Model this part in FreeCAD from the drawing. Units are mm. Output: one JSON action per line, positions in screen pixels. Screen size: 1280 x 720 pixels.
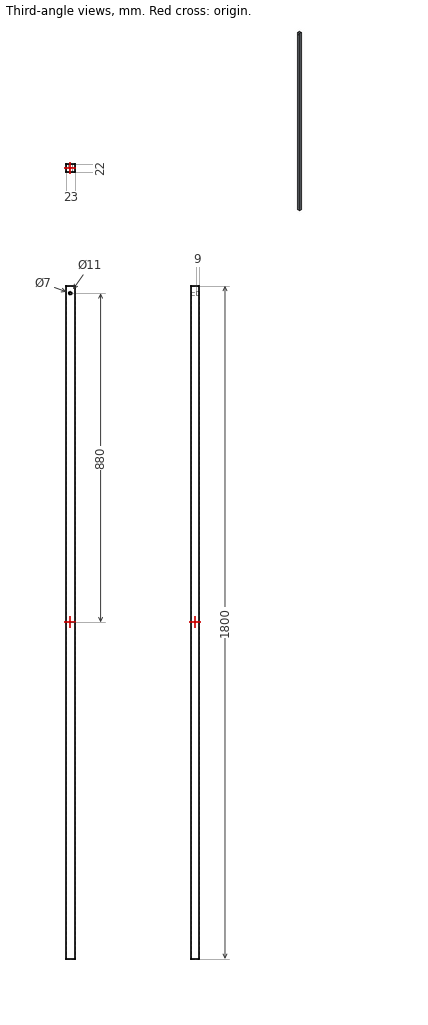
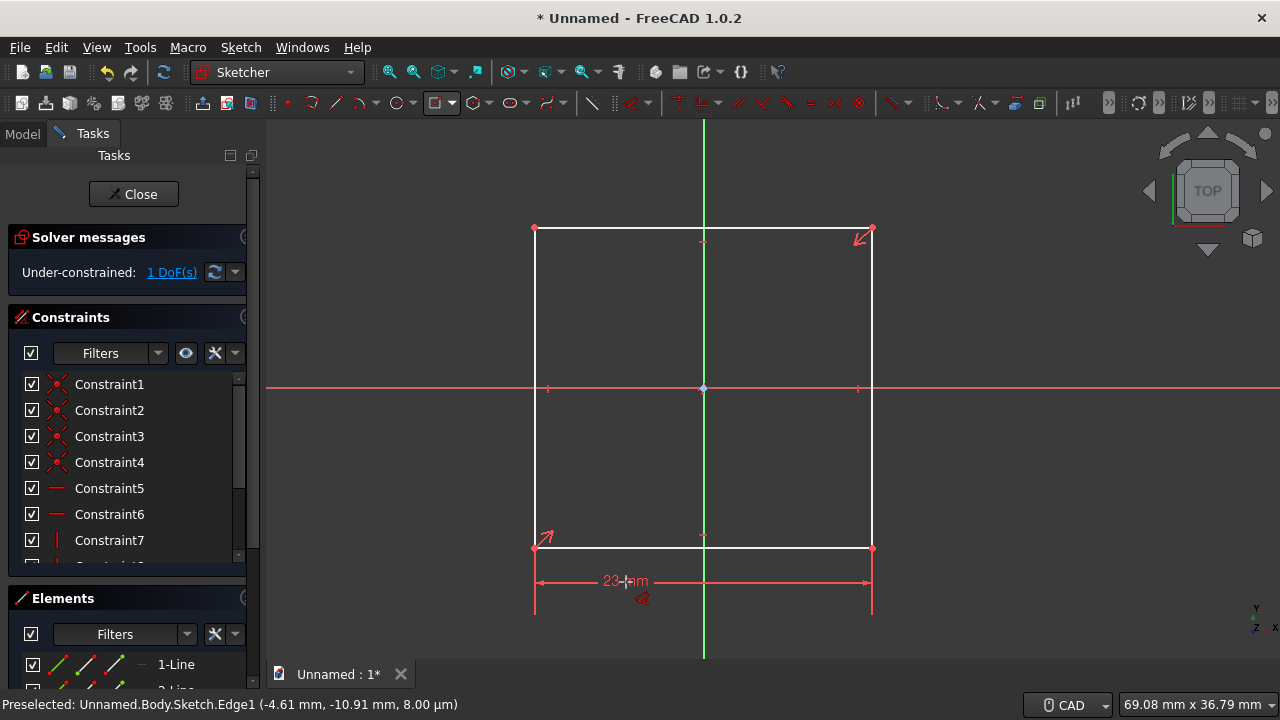
{"action": "left_click", "coordinate": [872, 452]}
{"action": "left_click", "coordinate": [906, 314]}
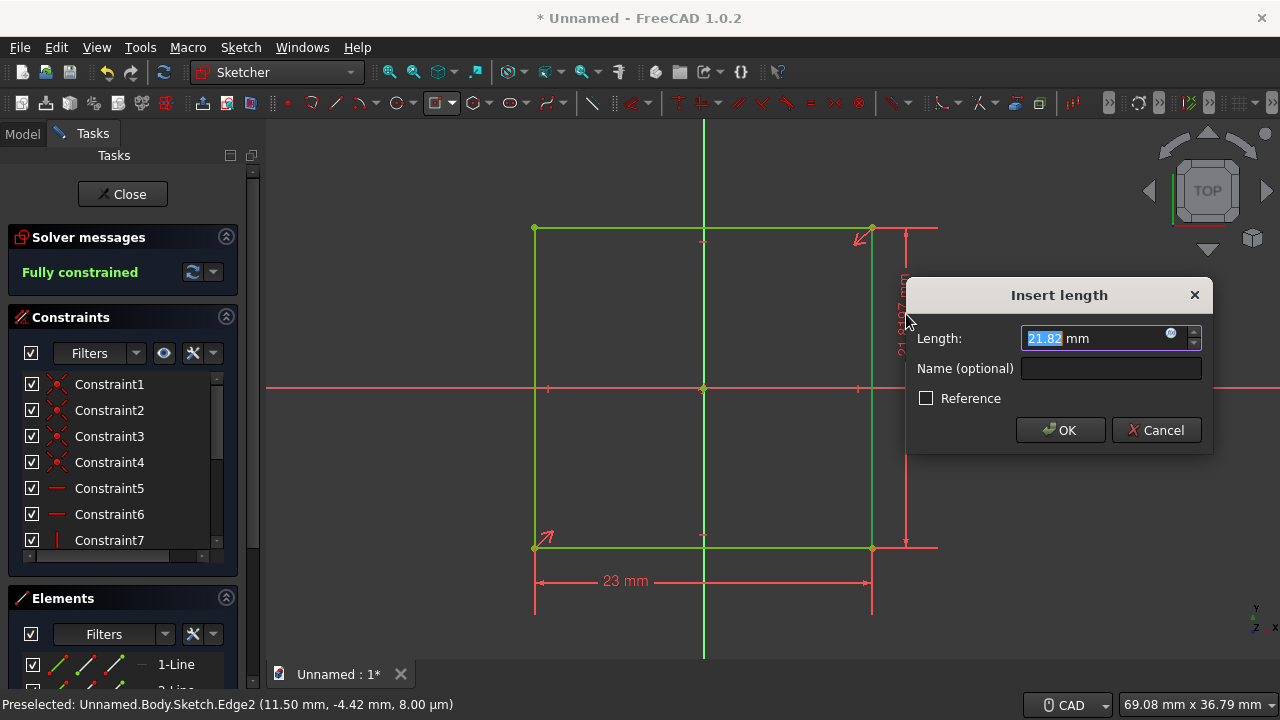
{"action": "type", "text": "22"}
{"action": "key", "text": "Return"}
{"action": "key", "text": "Escape"}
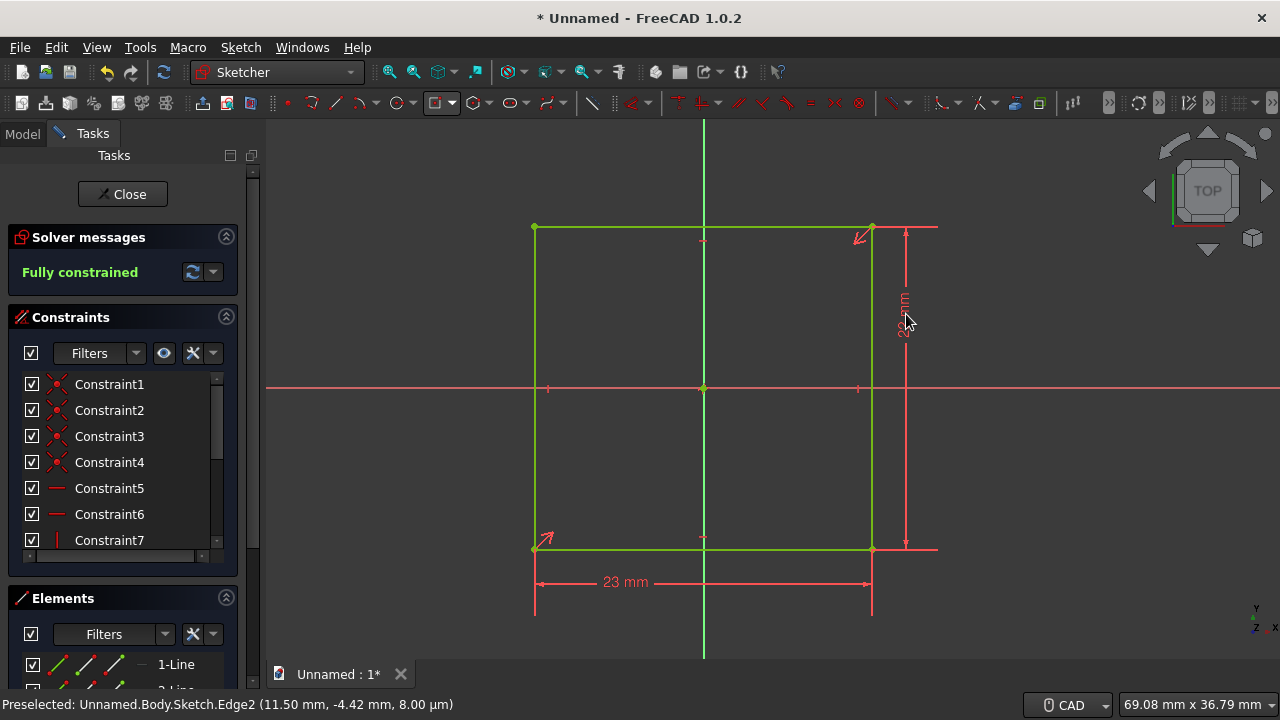
{"action": "left_click", "coordinate": [123, 194]}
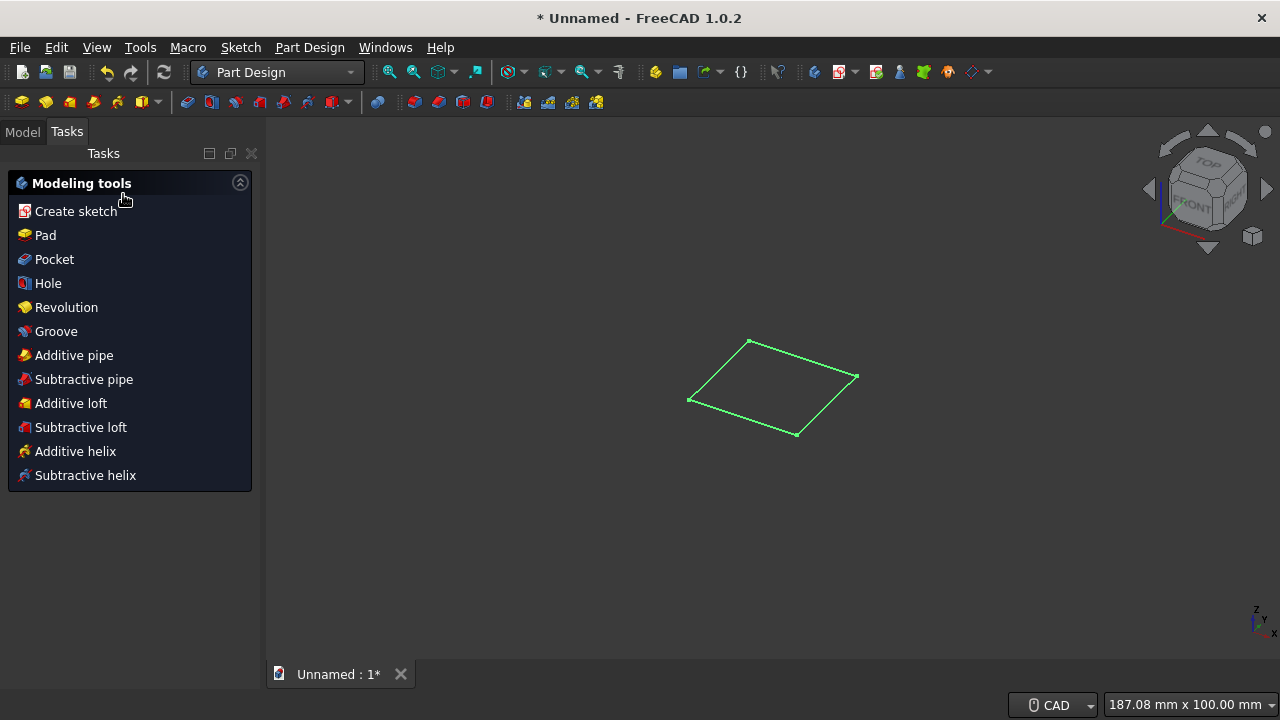
{"action": "left_click", "coordinate": [22, 102]}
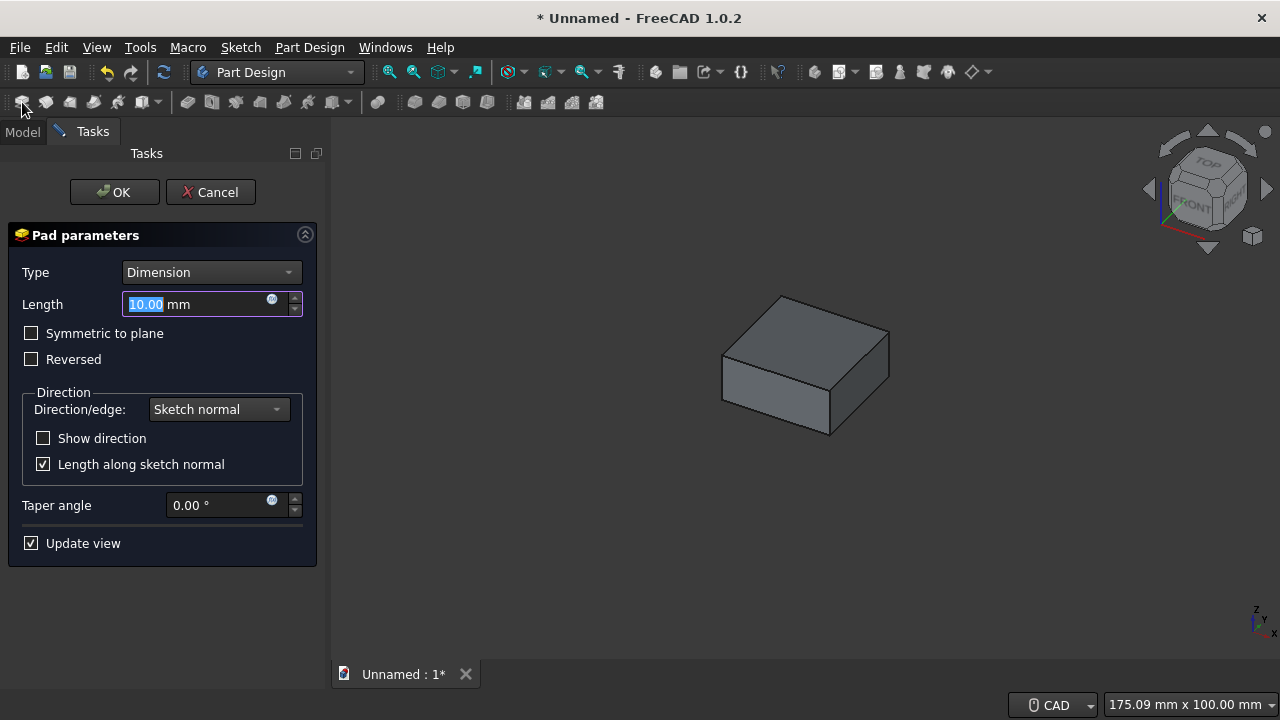
{"action": "type", "text": "1800"}
{"action": "key", "text": "Tab"}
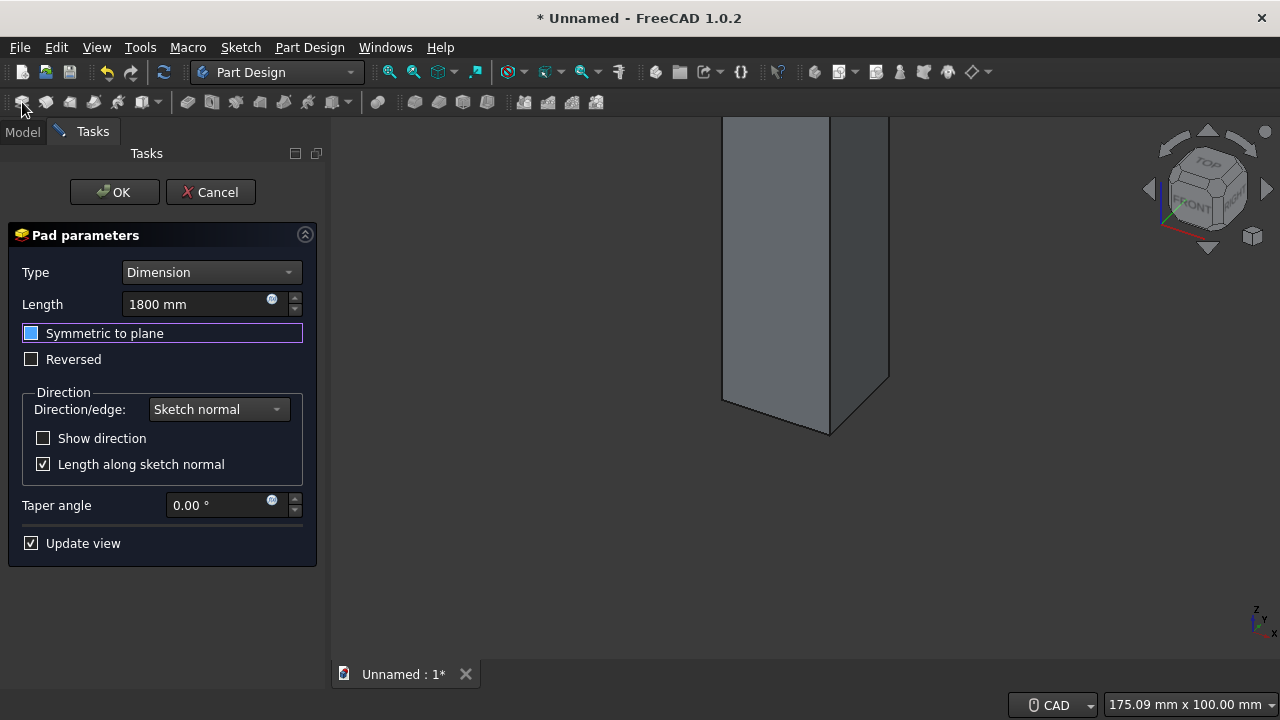
{"action": "left_click", "coordinate": [30, 333]}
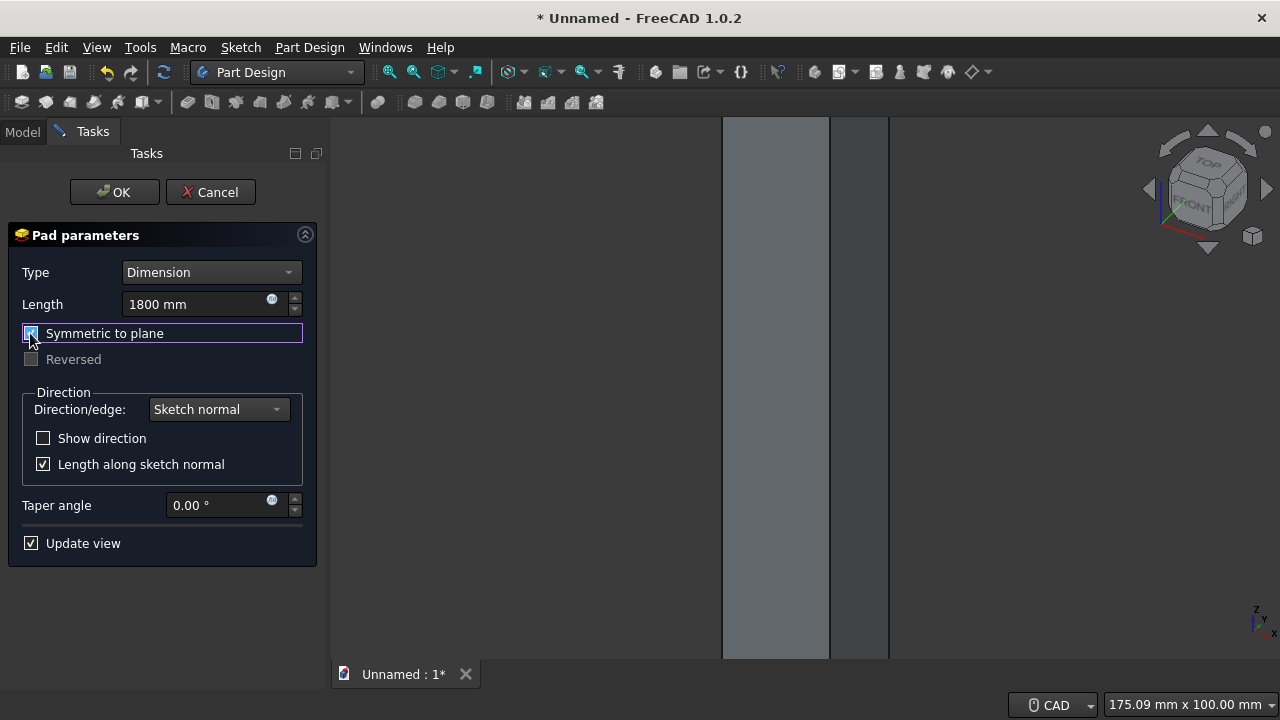
{"action": "left_click", "coordinate": [115, 192]}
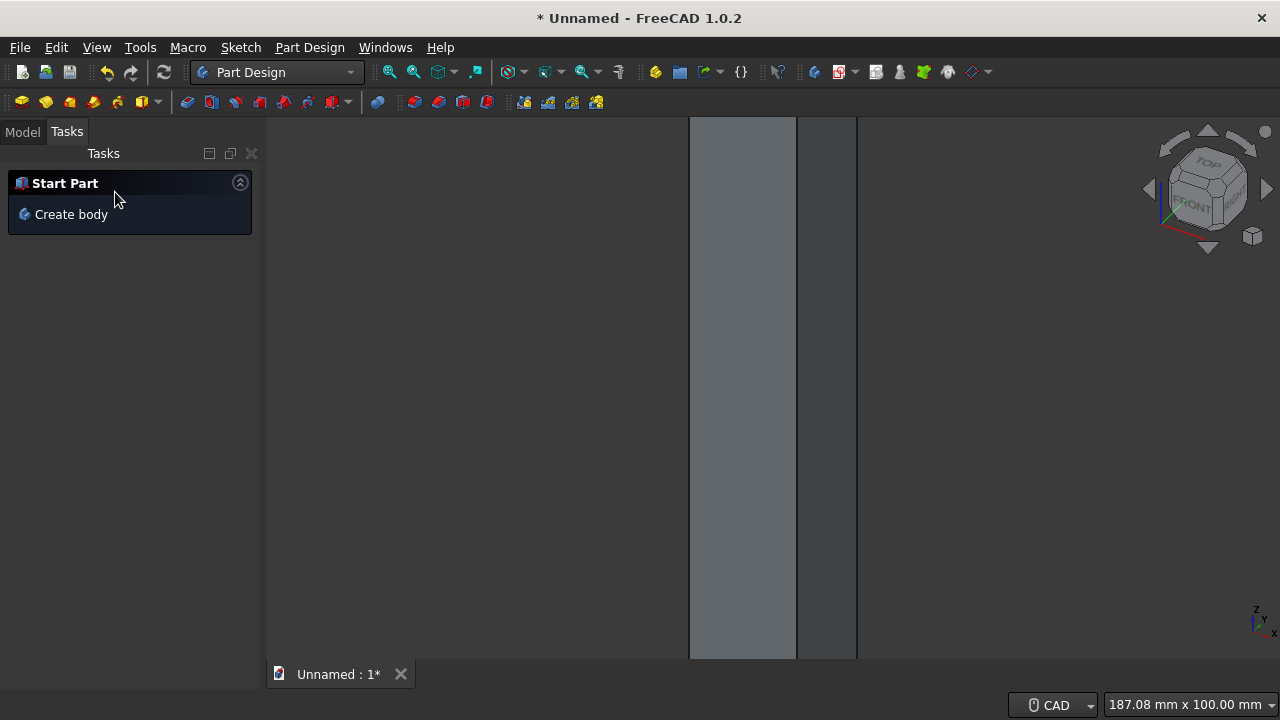
{"action": "left_click", "coordinate": [390, 72]}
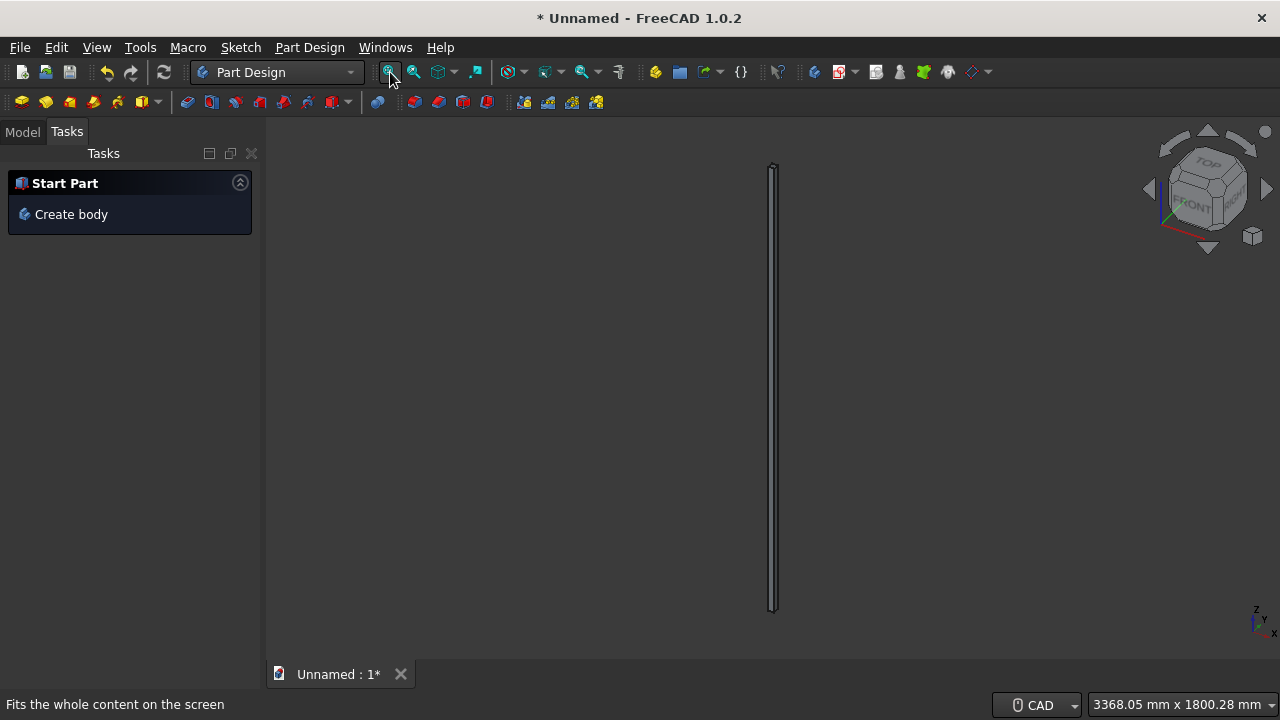
{"action": "key", "text": "4"}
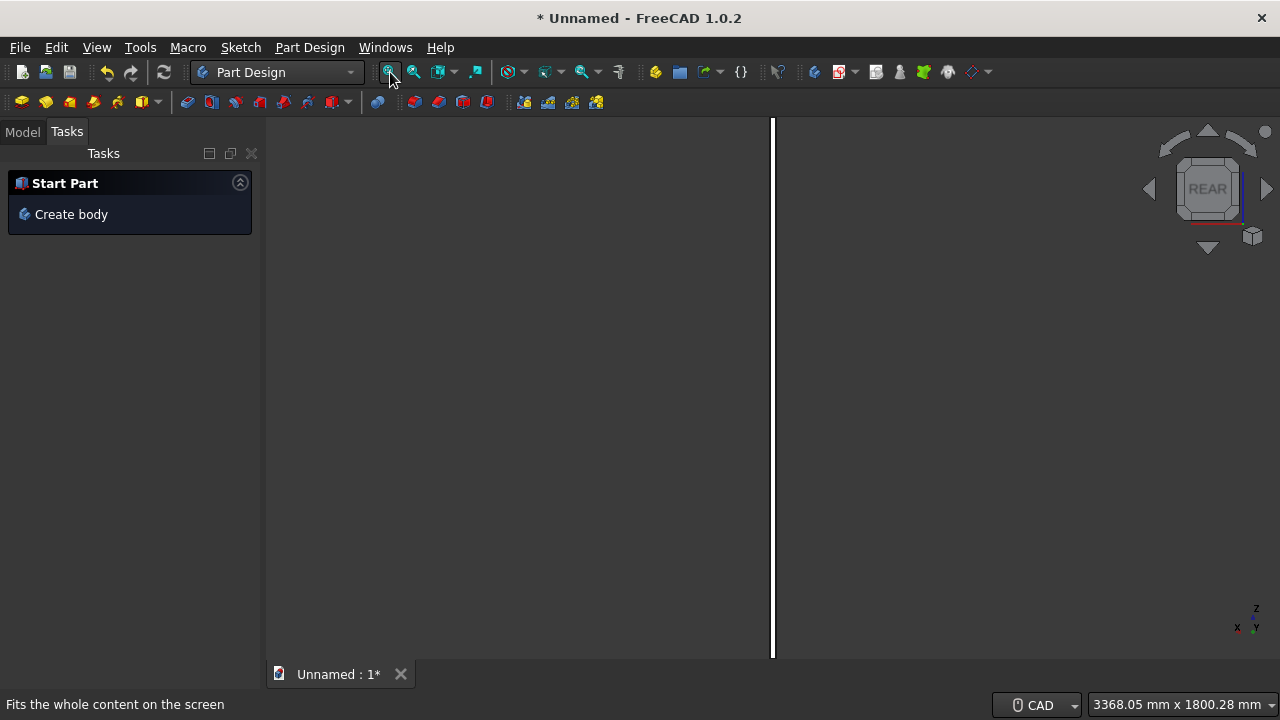
{"action": "left_click", "coordinate": [390, 72]}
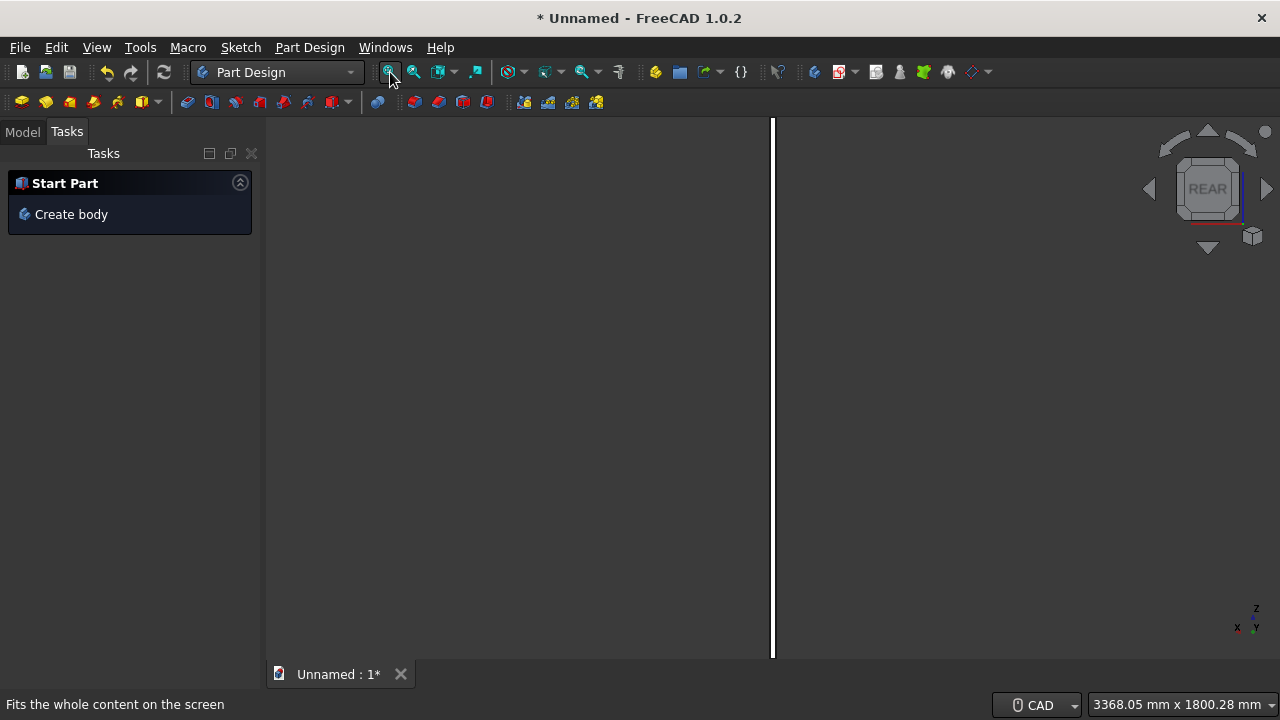
{"action": "scroll", "coordinate": [773, 155], "scroll_direction": "up", "scroll_amount": 7}